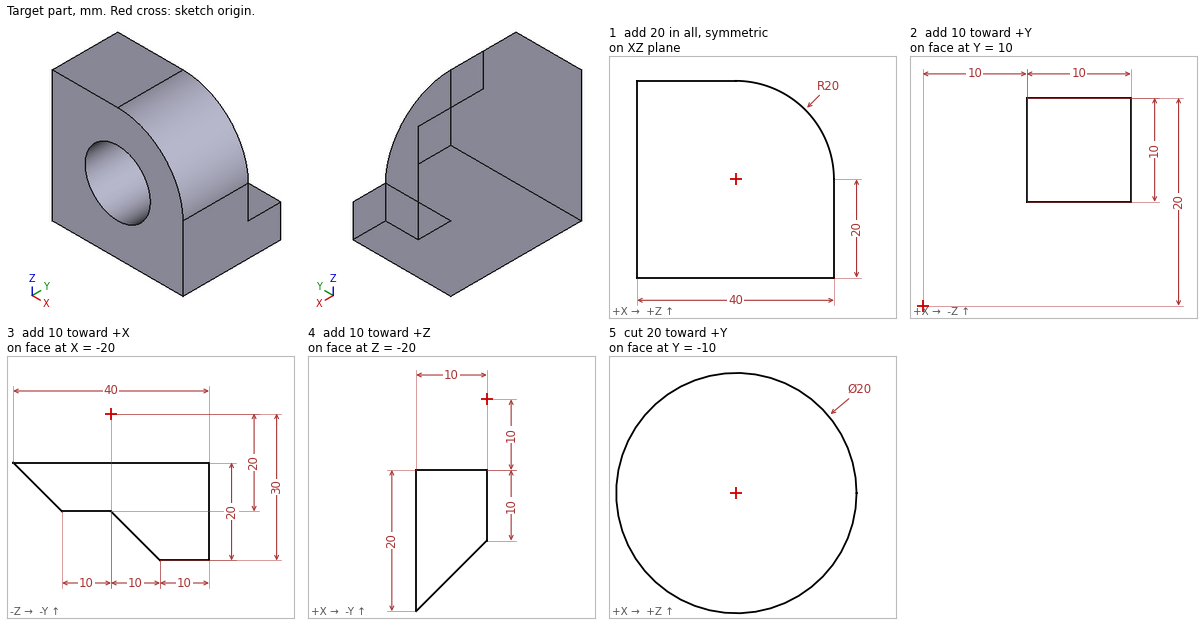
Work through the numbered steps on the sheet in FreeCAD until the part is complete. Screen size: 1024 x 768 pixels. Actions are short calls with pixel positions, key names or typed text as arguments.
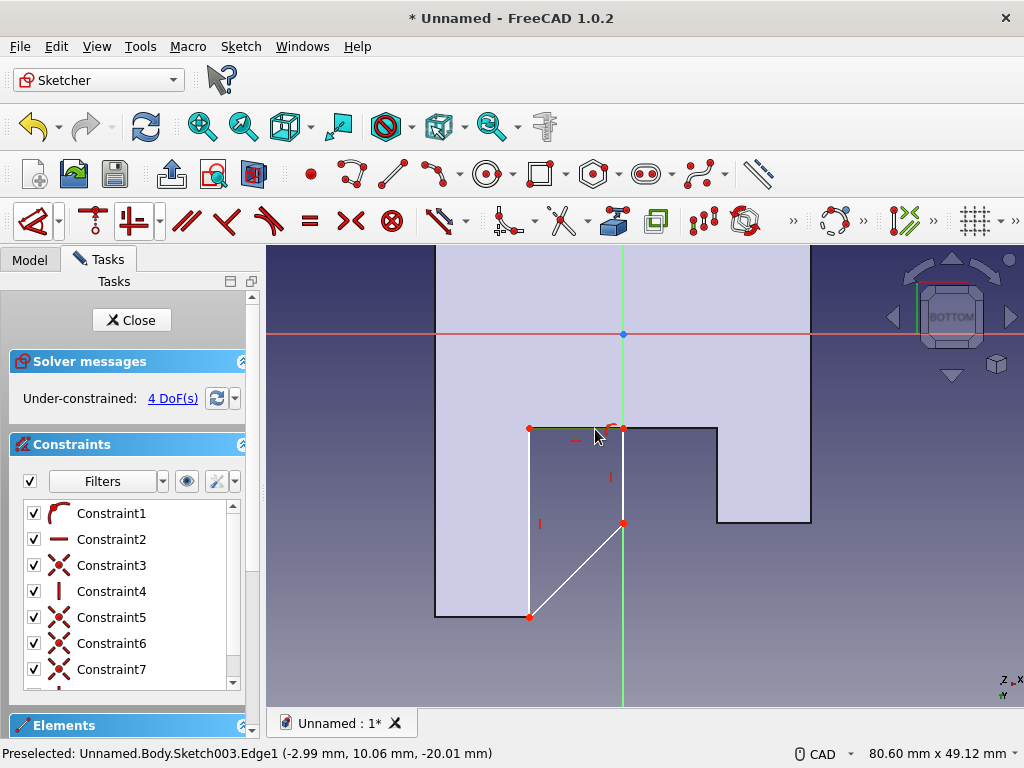
key(l)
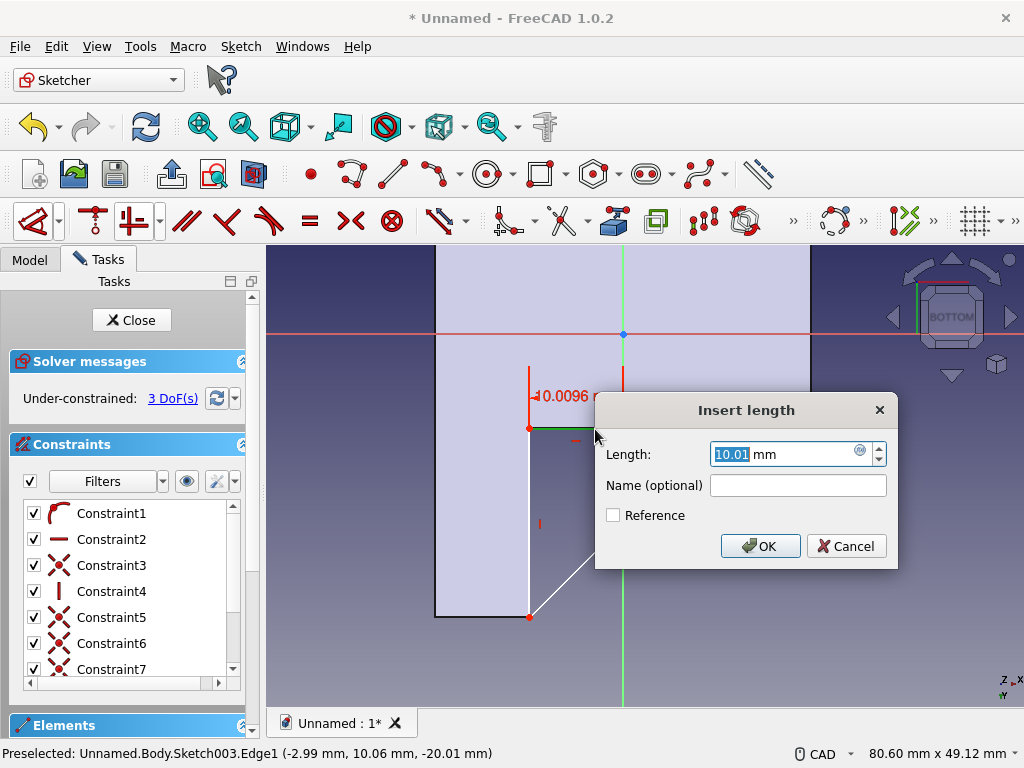
text(10)
key(Return)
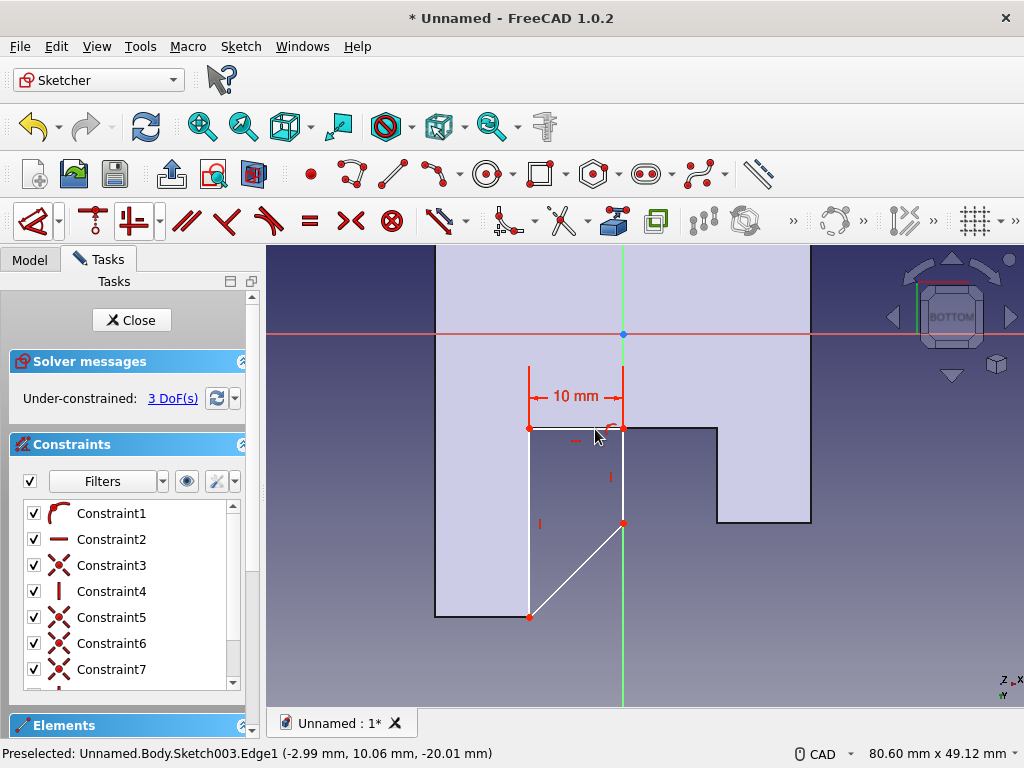
click(529, 486)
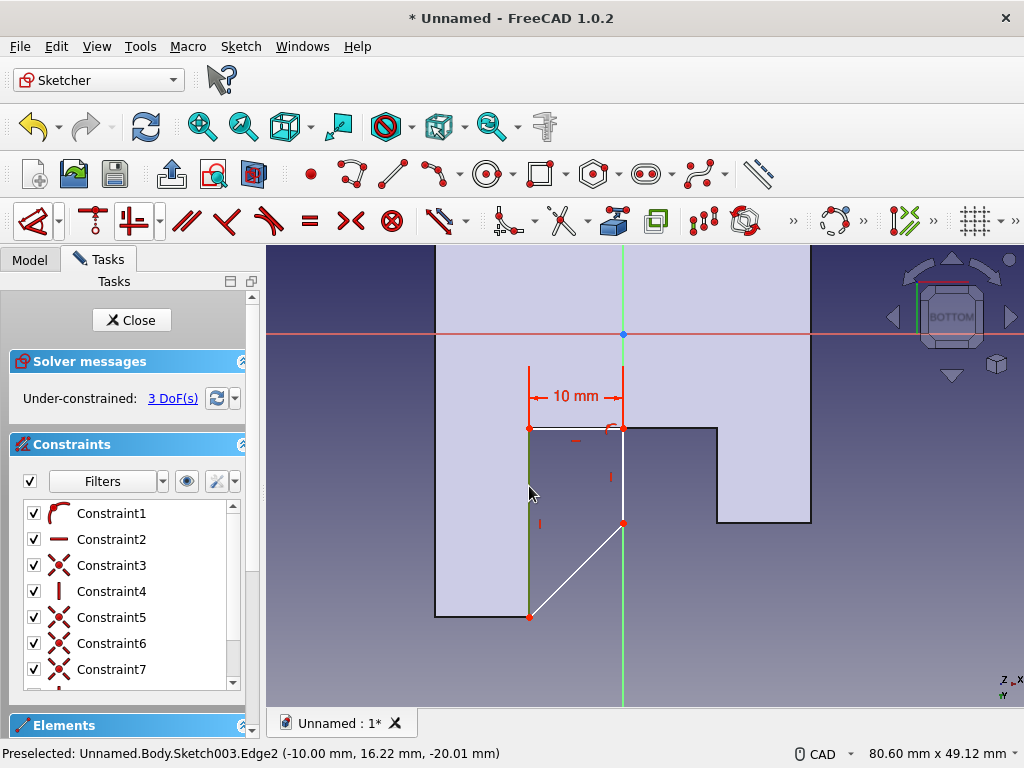
click(58, 222)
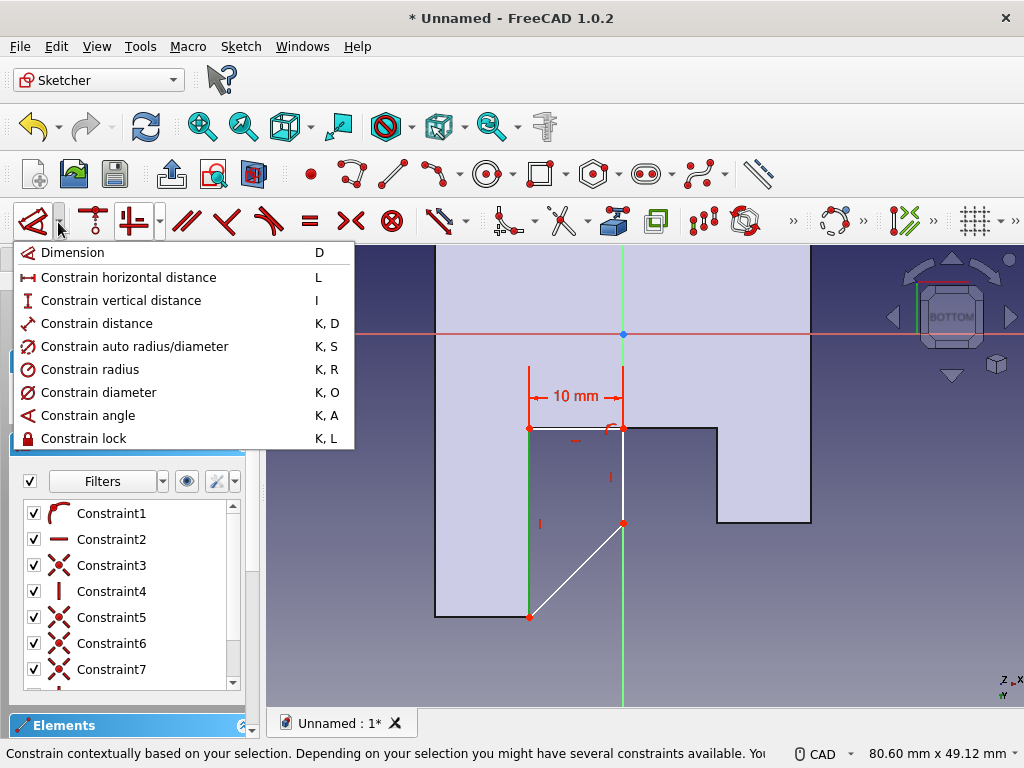
click(184, 300)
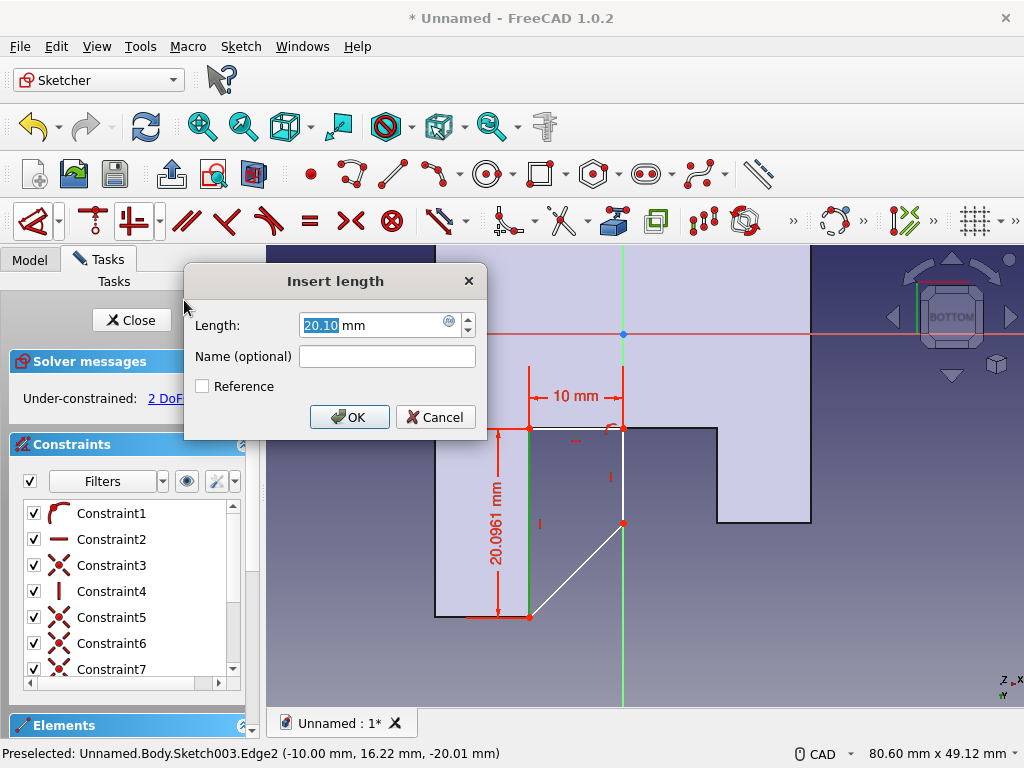
text(20)
key(Return)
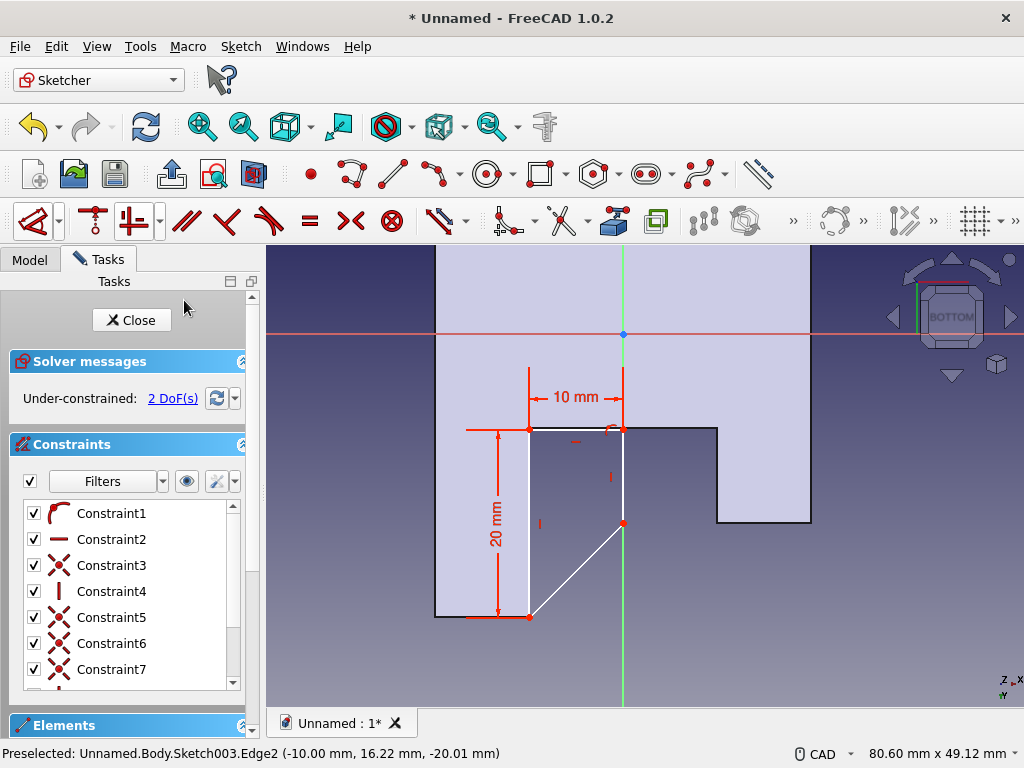
click(623, 496)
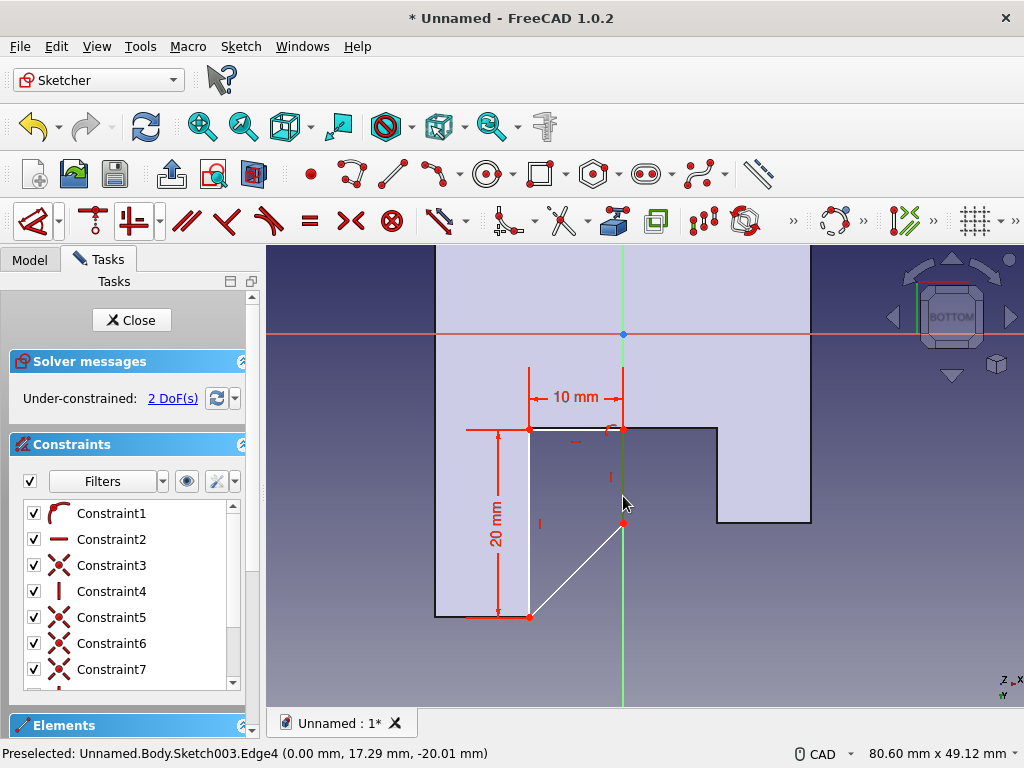
click(58, 222)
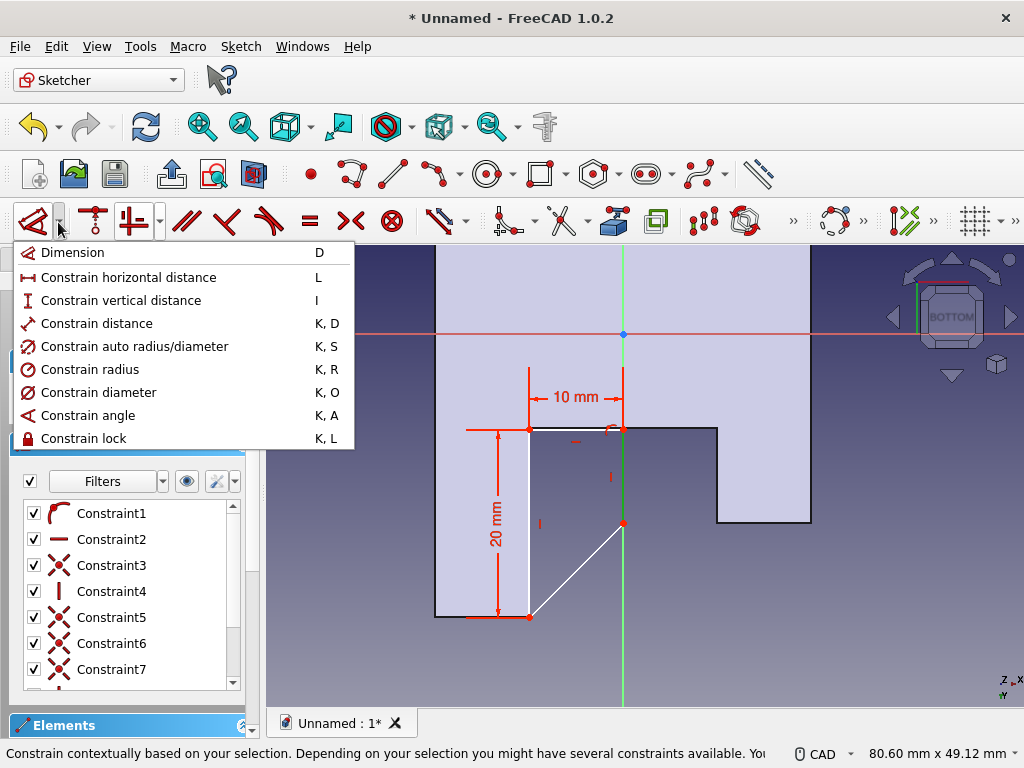
click(184, 300)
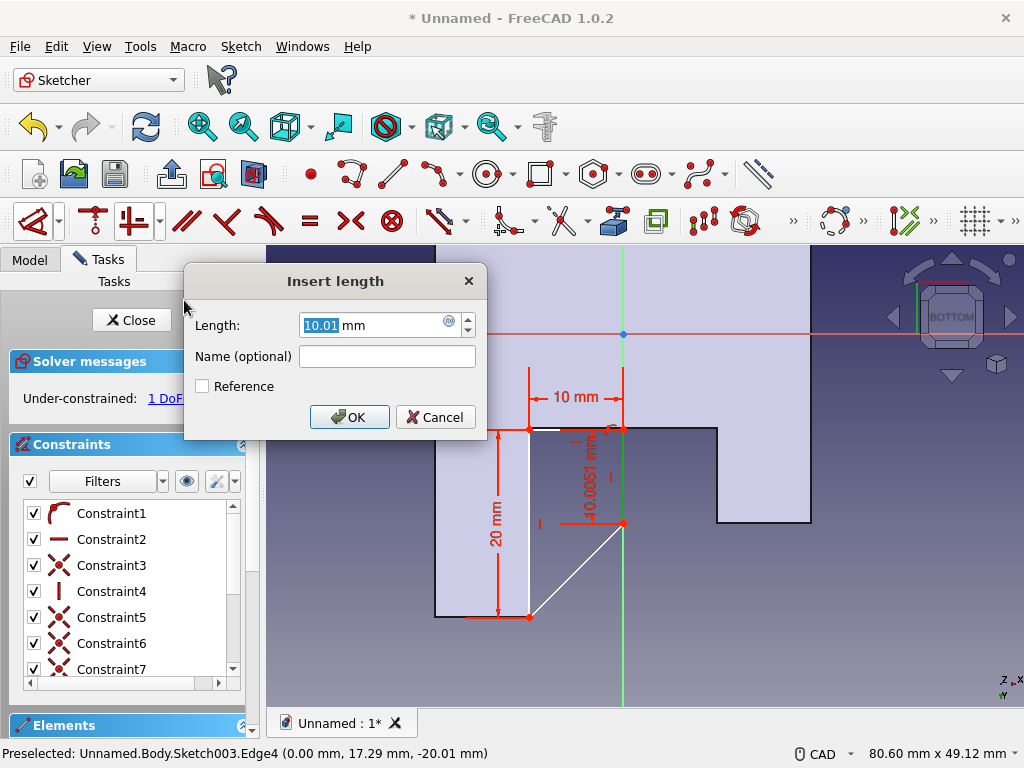
text(10)
key(Return)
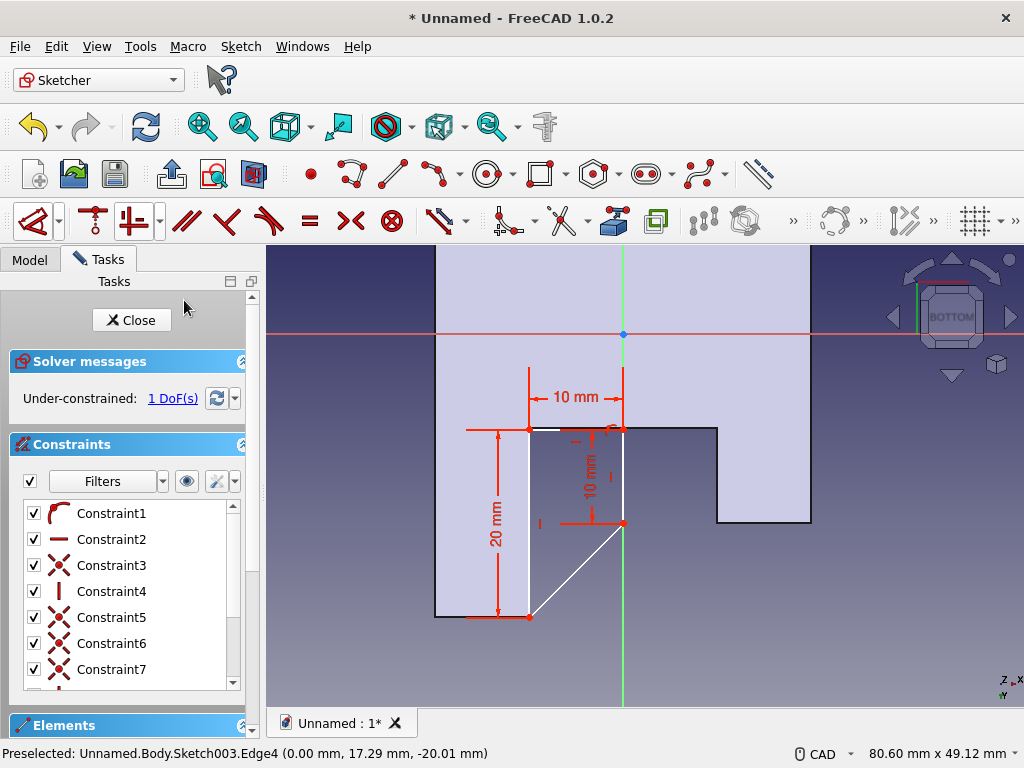
click(623, 430)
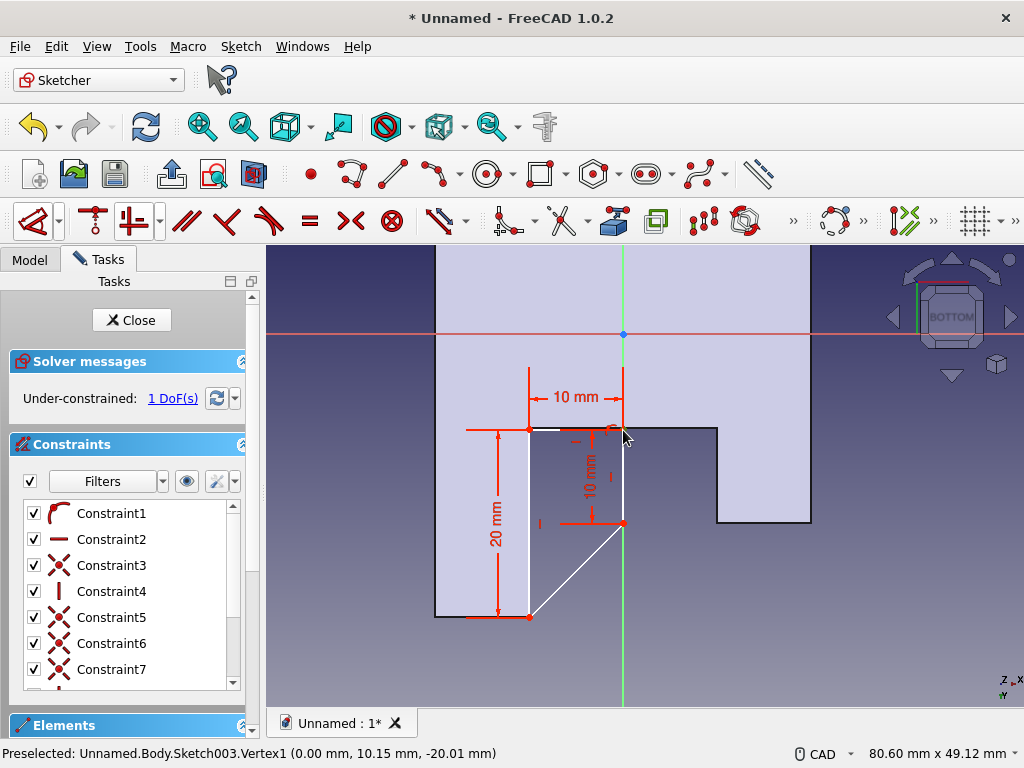
key(i)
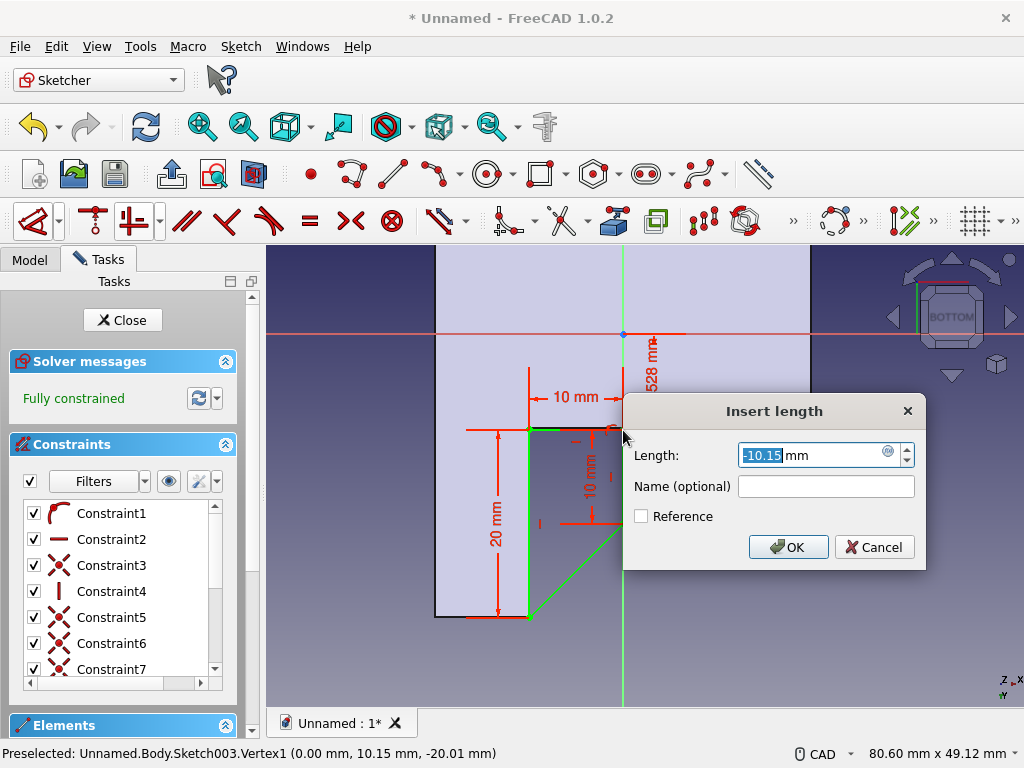
text(-10)
key(Return)